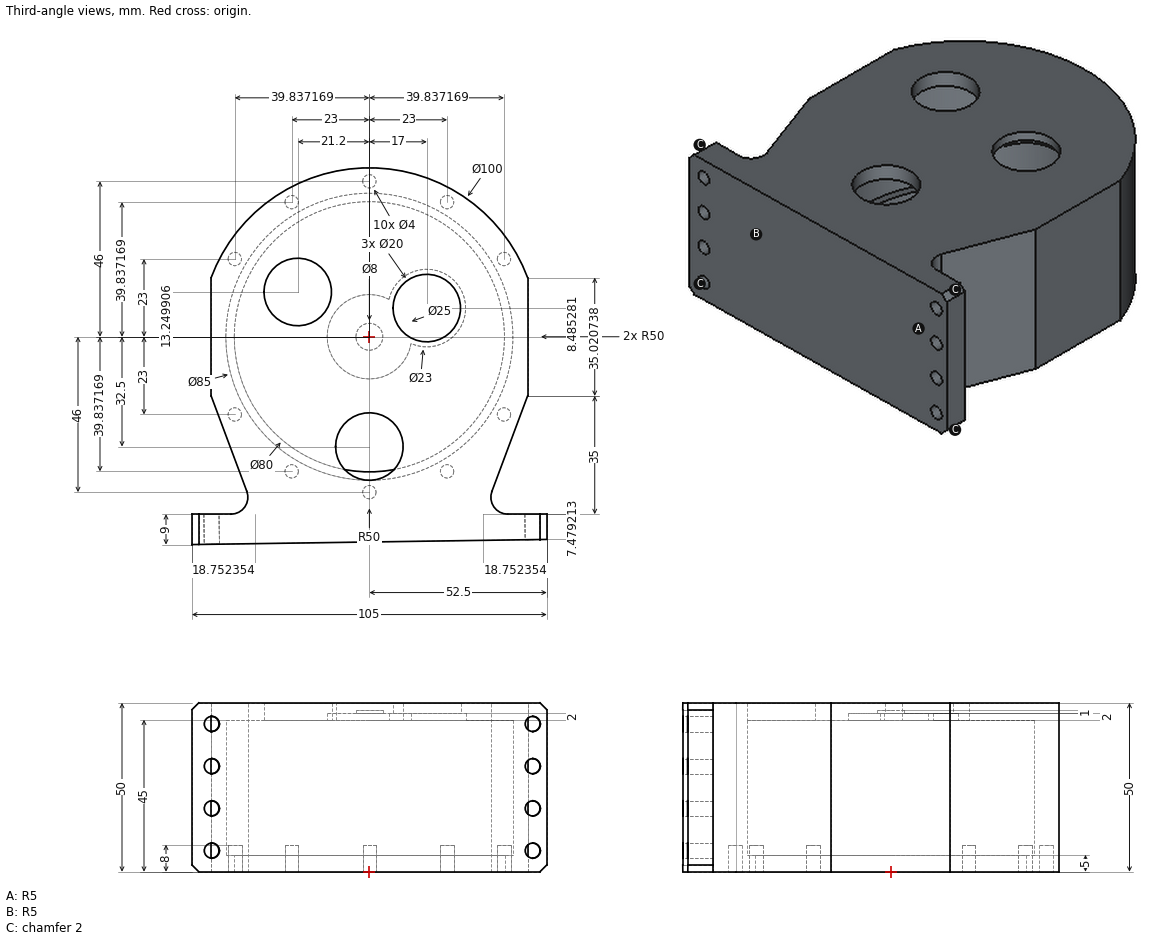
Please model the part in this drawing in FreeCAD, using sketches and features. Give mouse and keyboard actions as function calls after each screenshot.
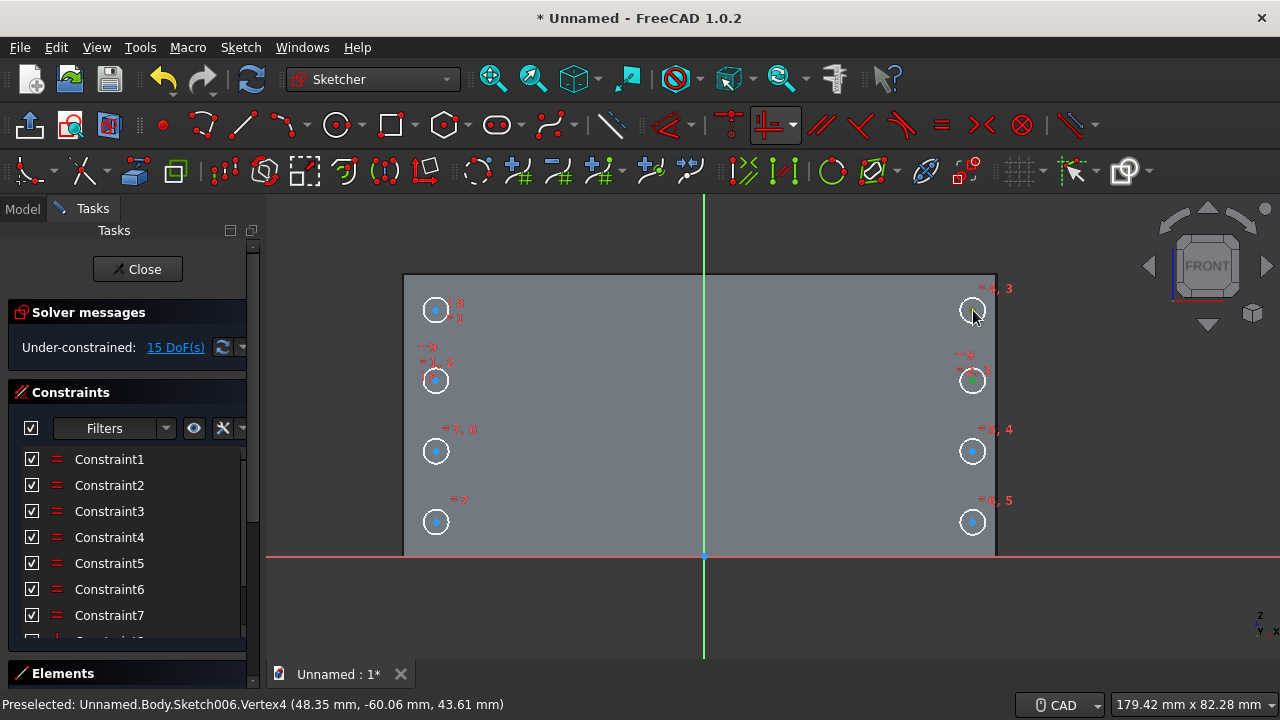
click(796, 126)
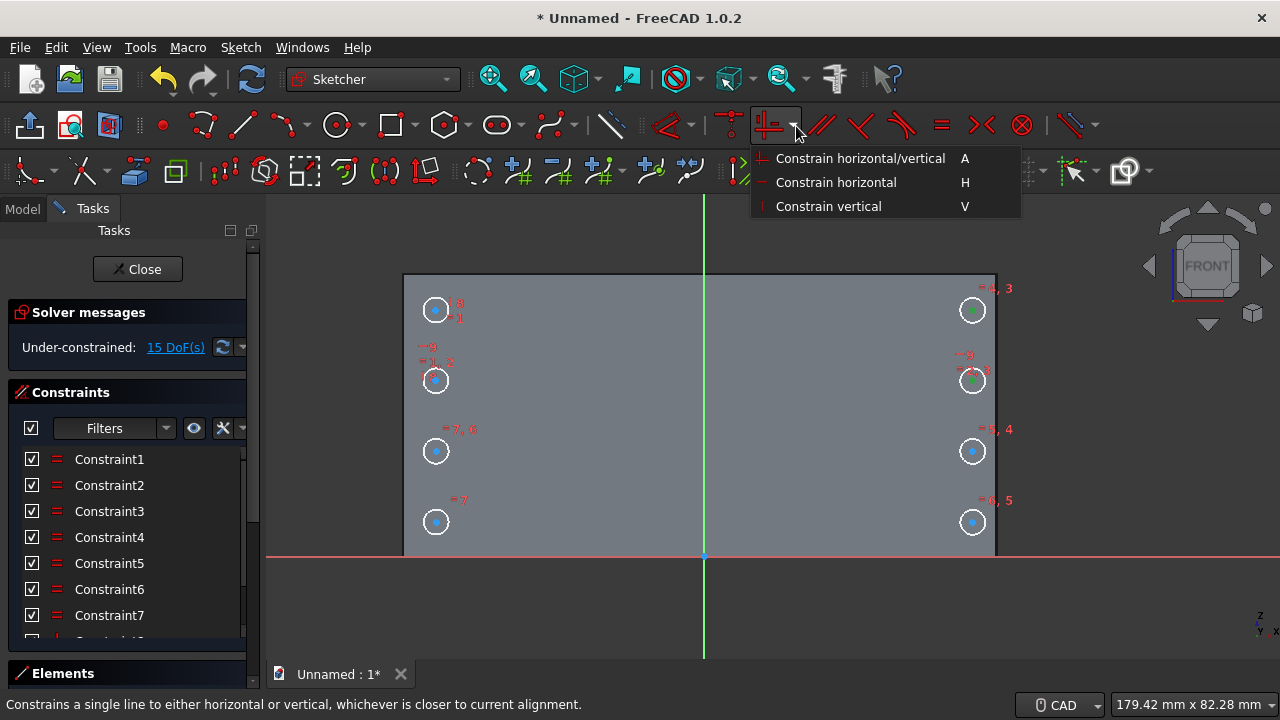
click(886, 206)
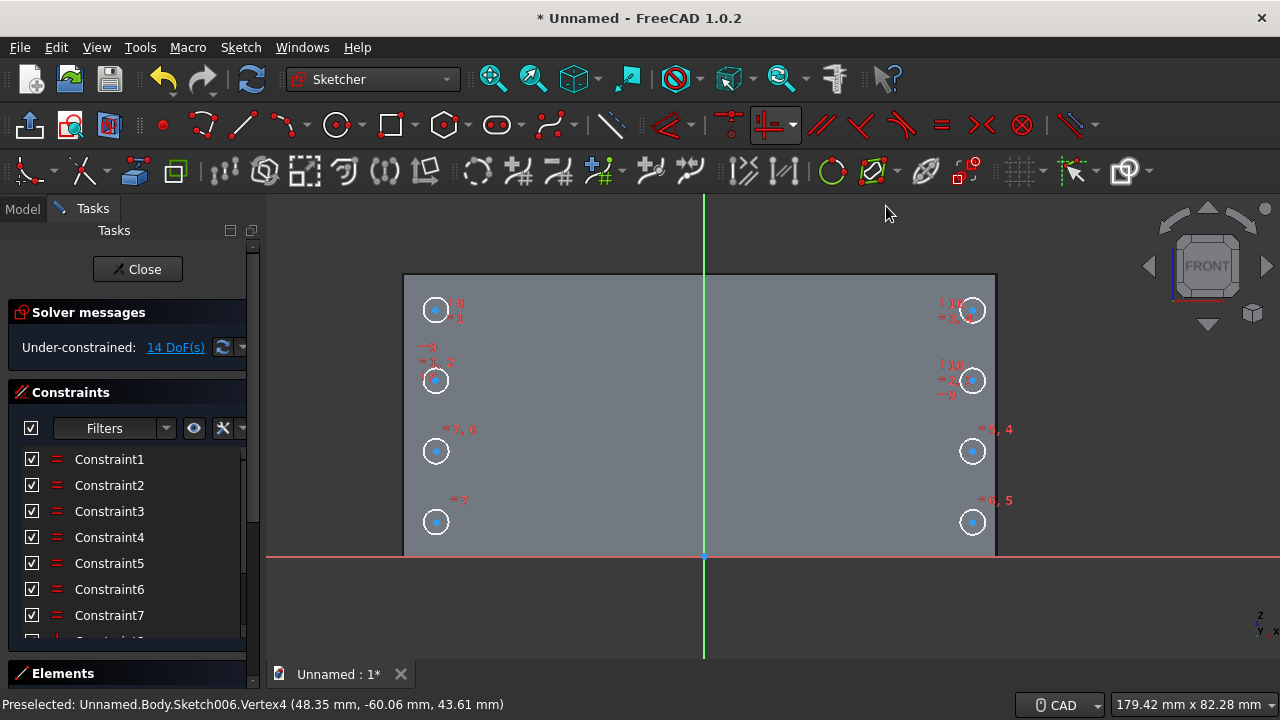
click(436, 310)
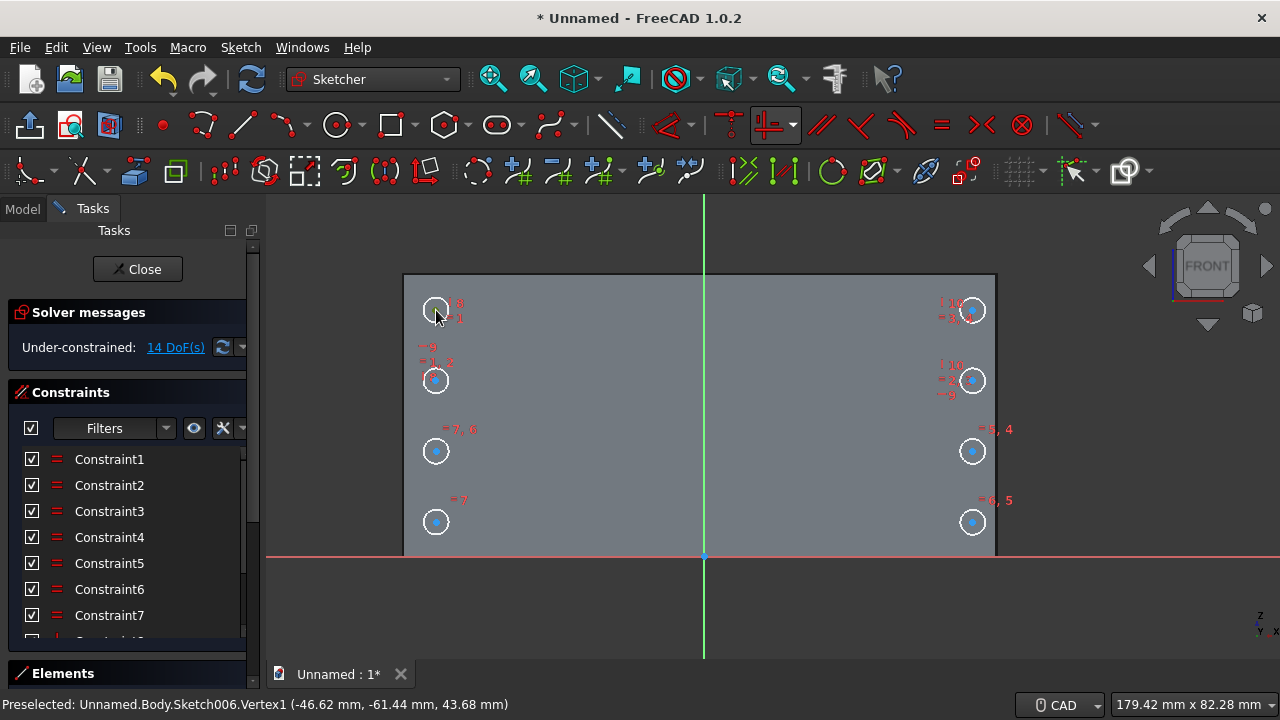
click(973, 310)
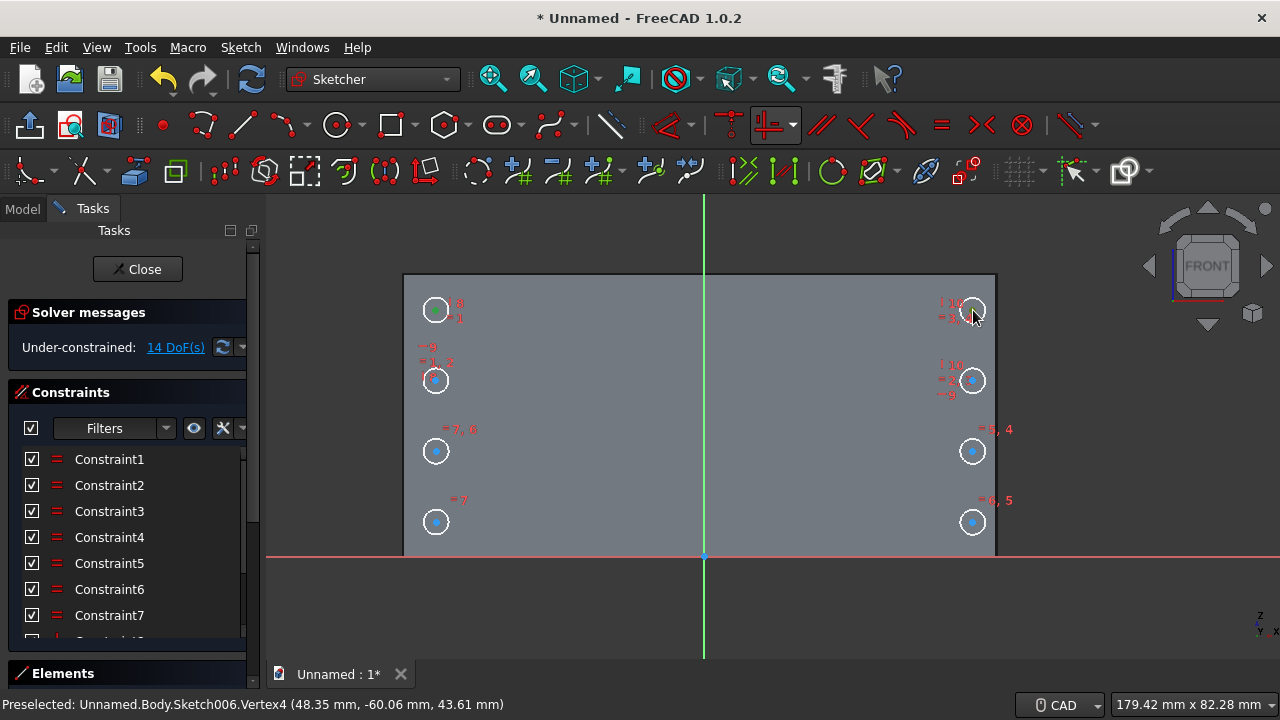
key(h)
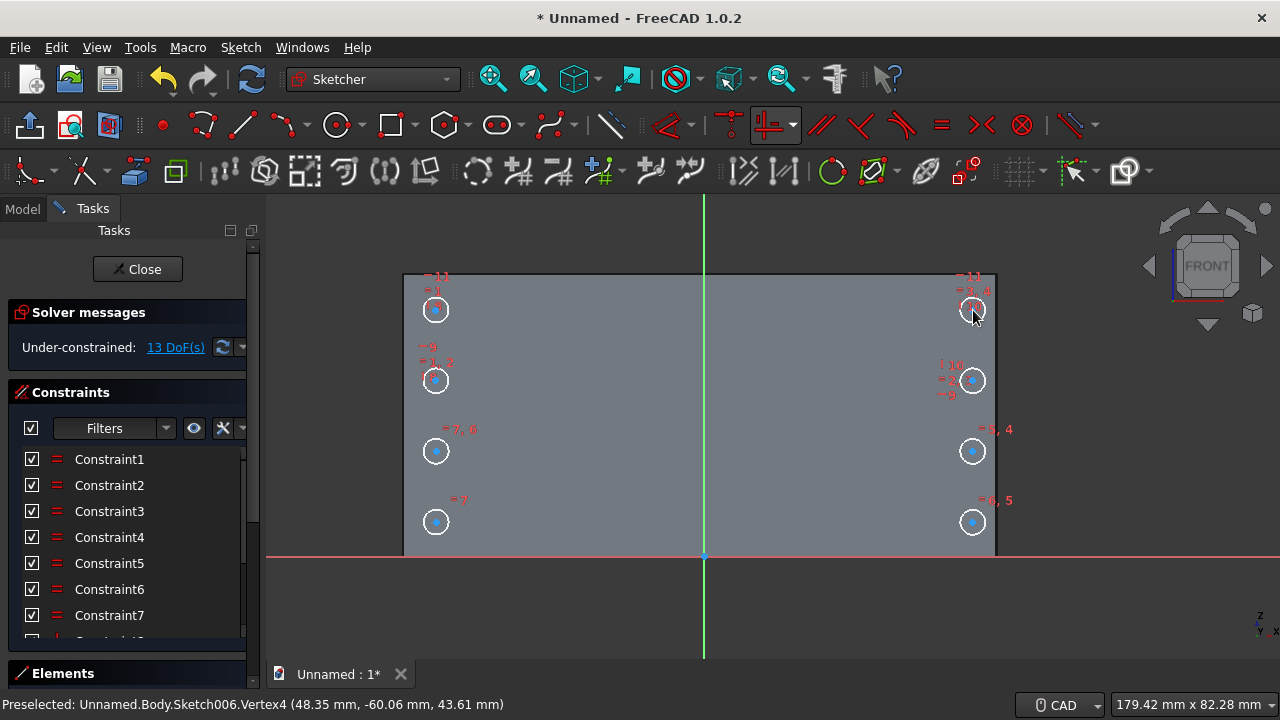
click(973, 381)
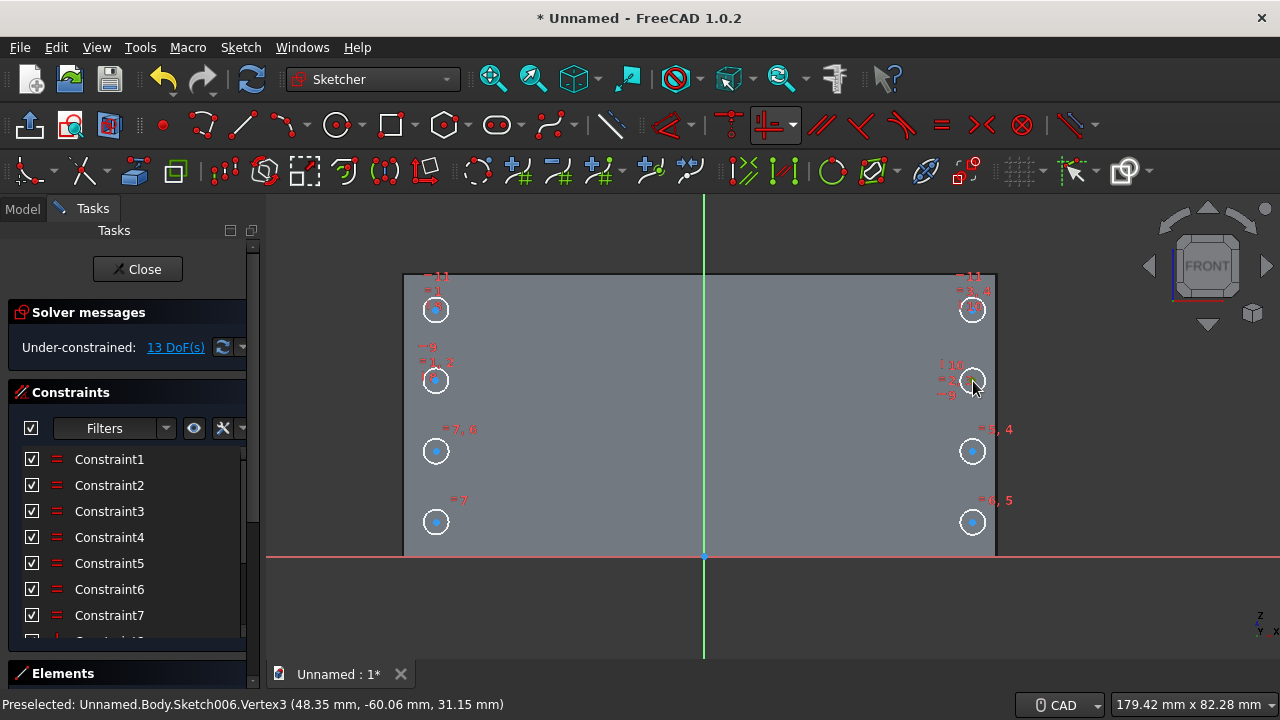
click(973, 451)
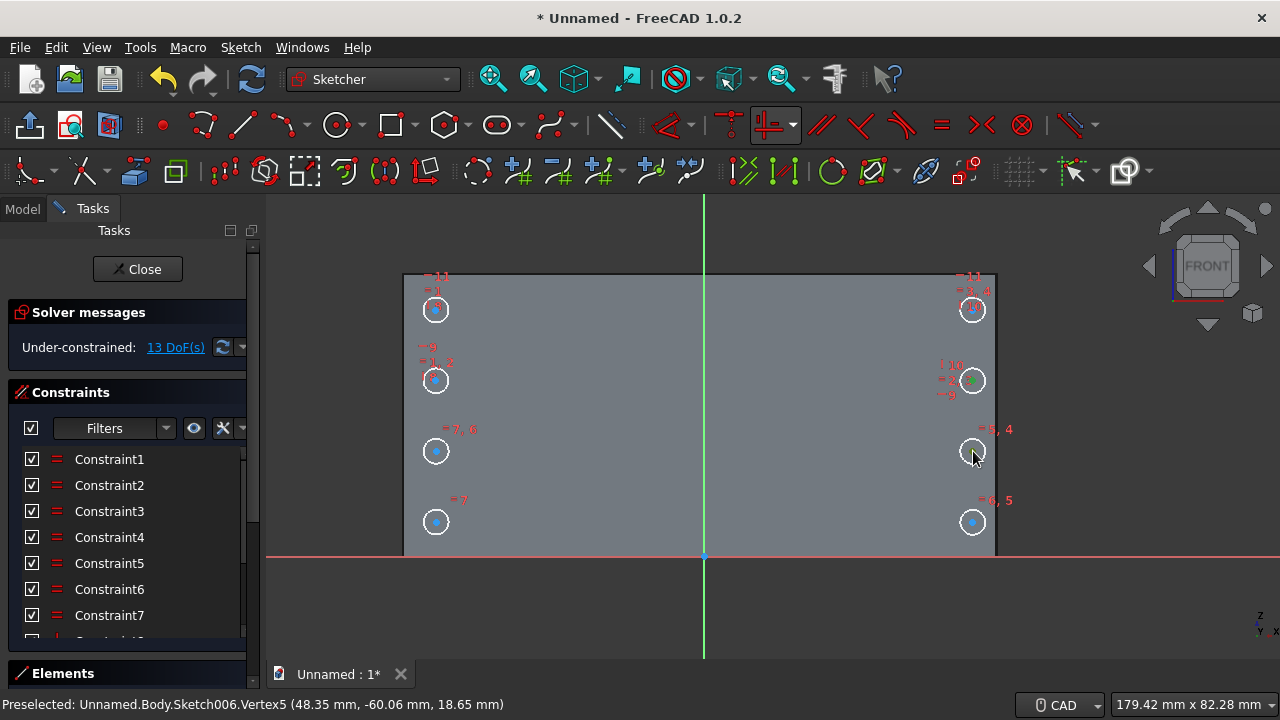
click(796, 126)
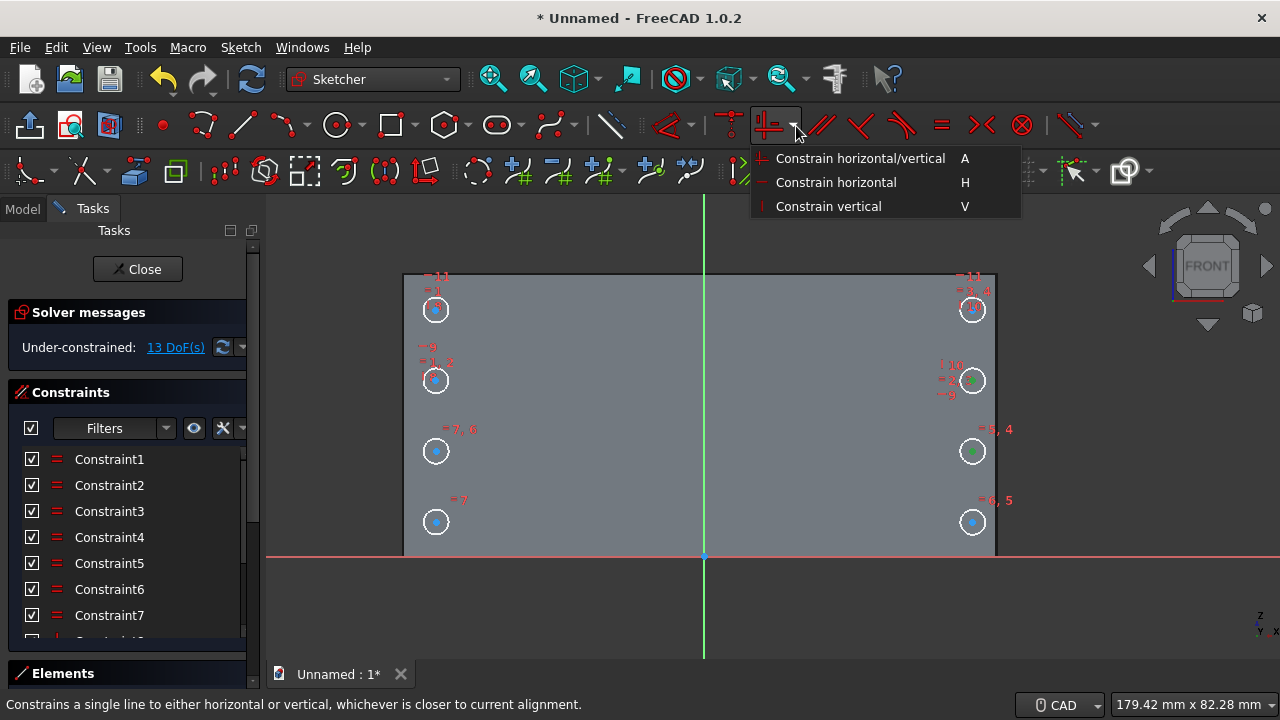
click(886, 206)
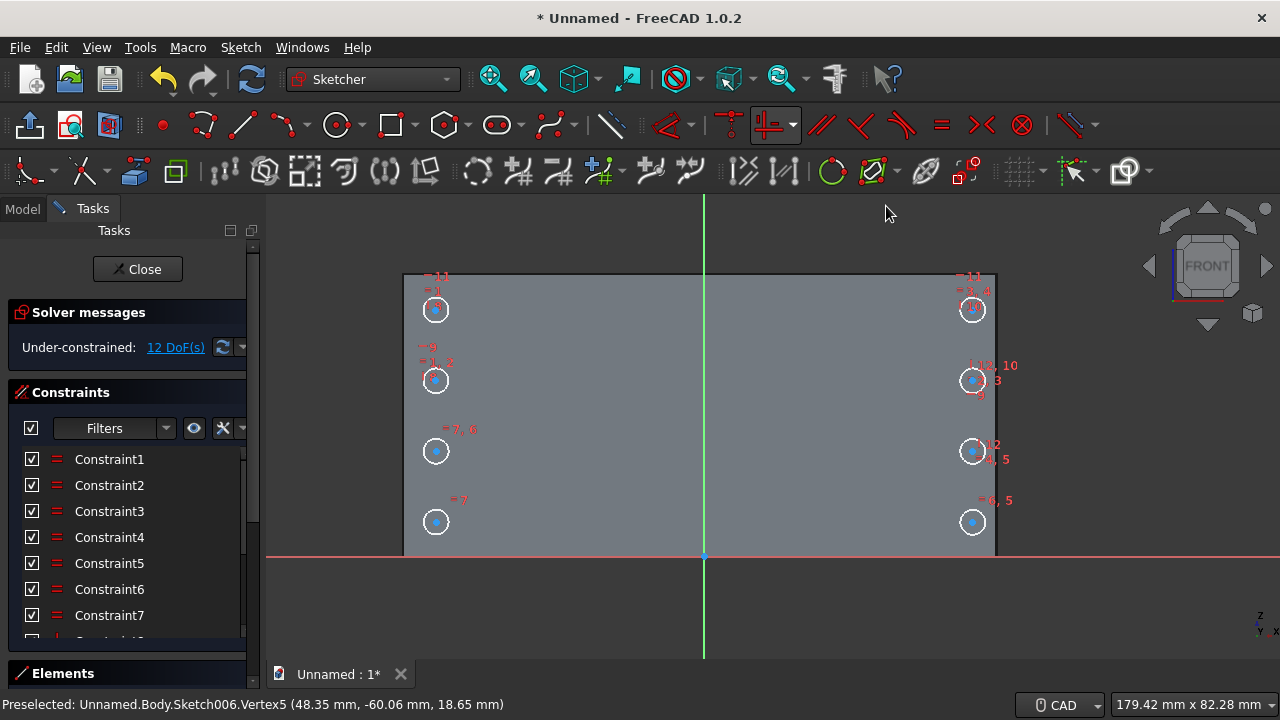
click(971, 453)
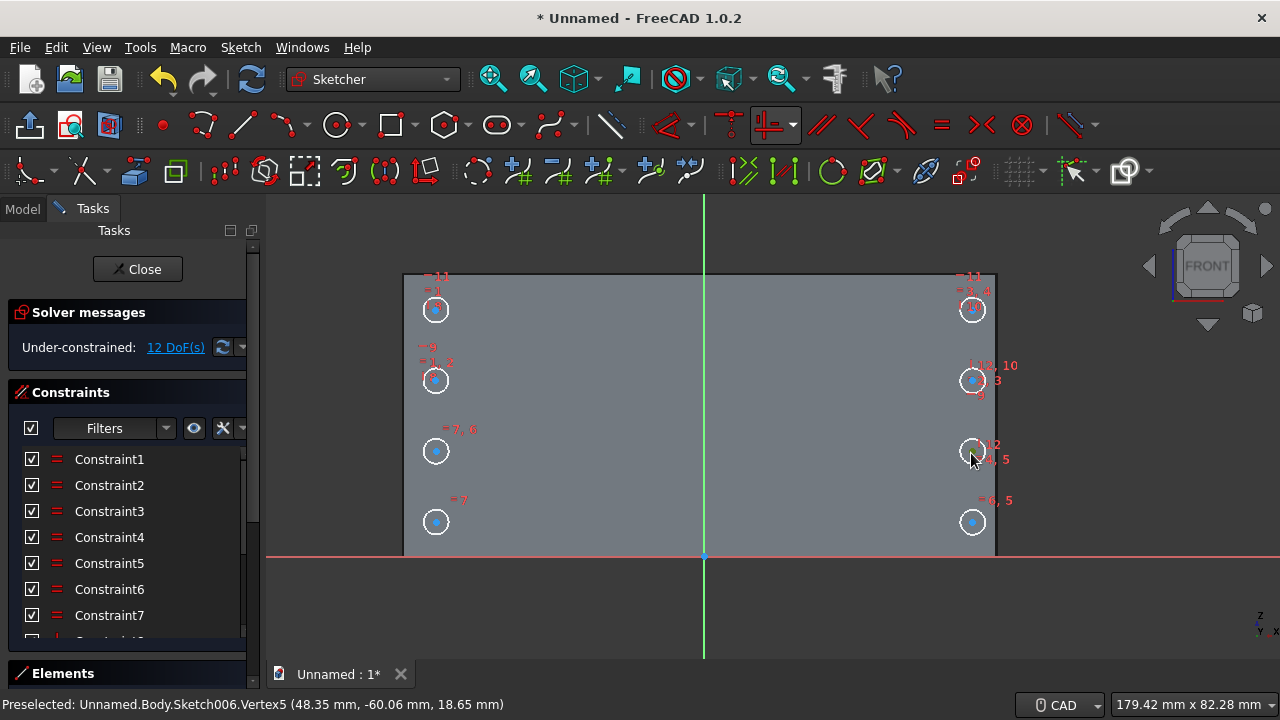
click(973, 522)